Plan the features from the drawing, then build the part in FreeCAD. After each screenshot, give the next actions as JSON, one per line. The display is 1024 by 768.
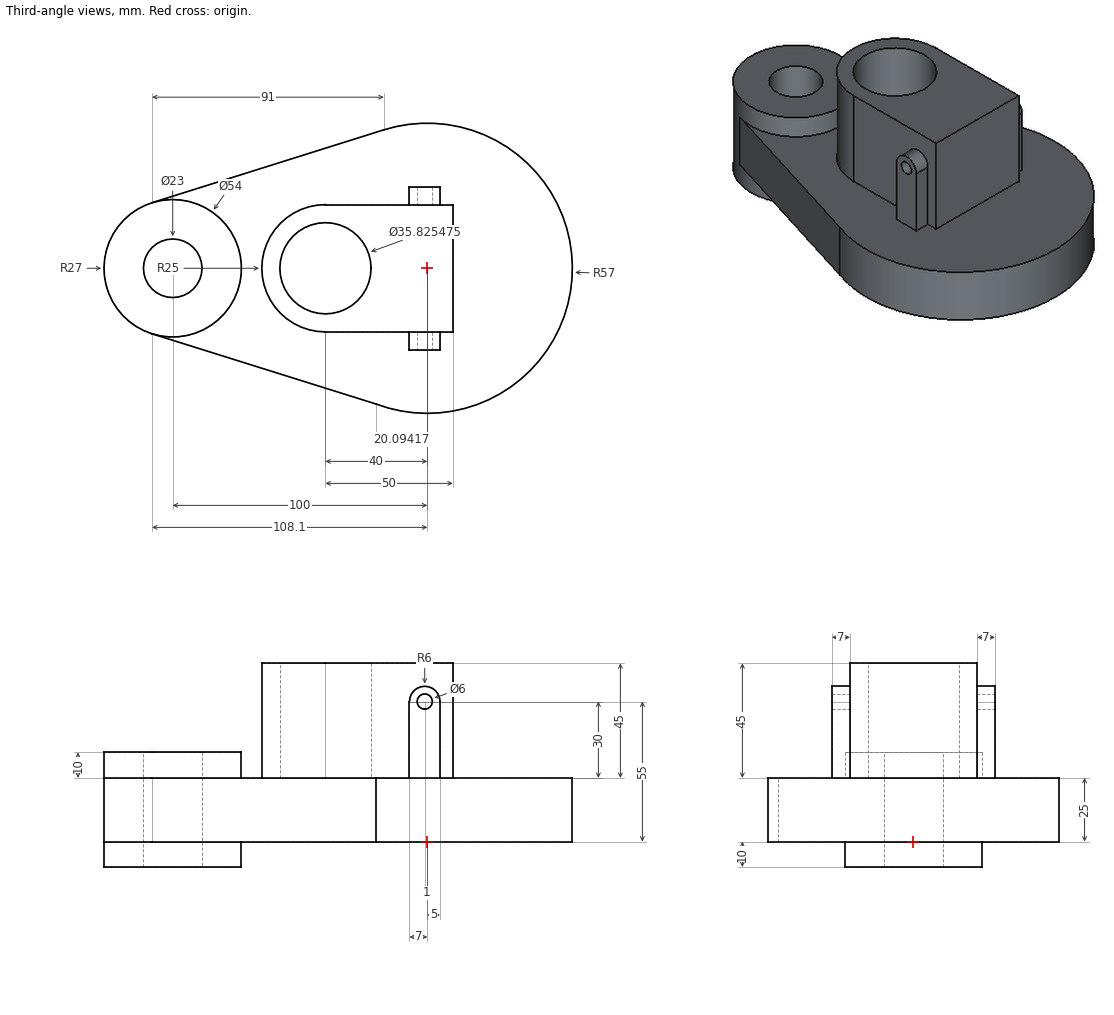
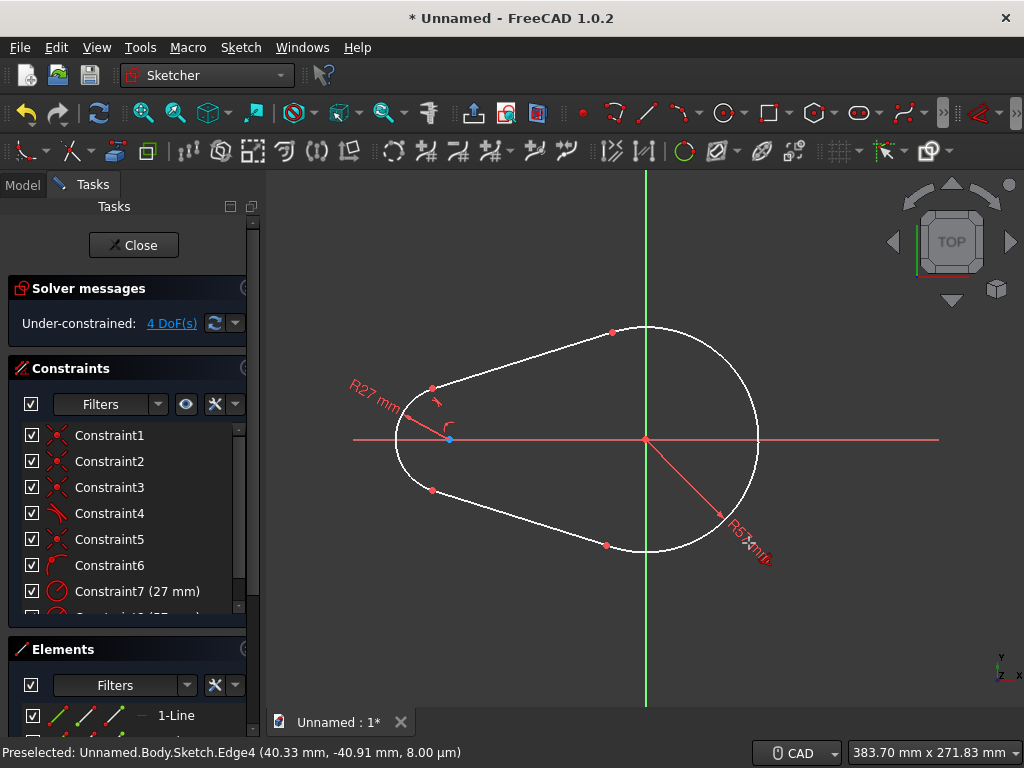
{"action": "left_click", "coordinate": [558, 349]}
{"action": "left_click", "coordinate": [523, 298]}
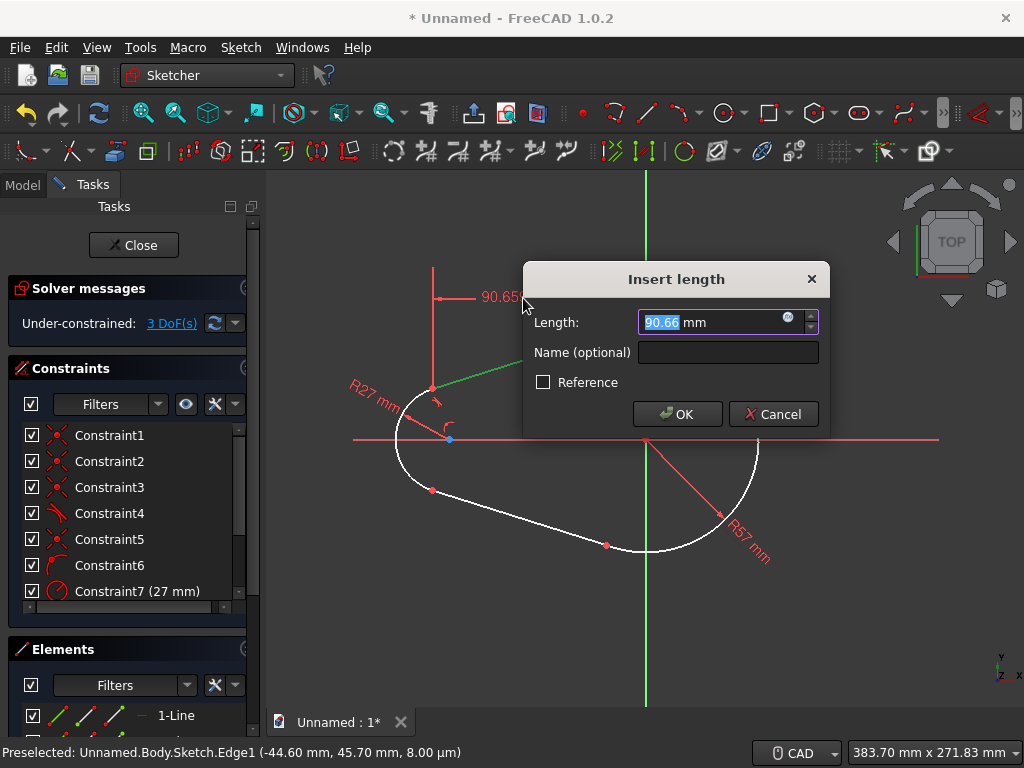
{"action": "type", "text": "91"}
{"action": "key", "text": "Return"}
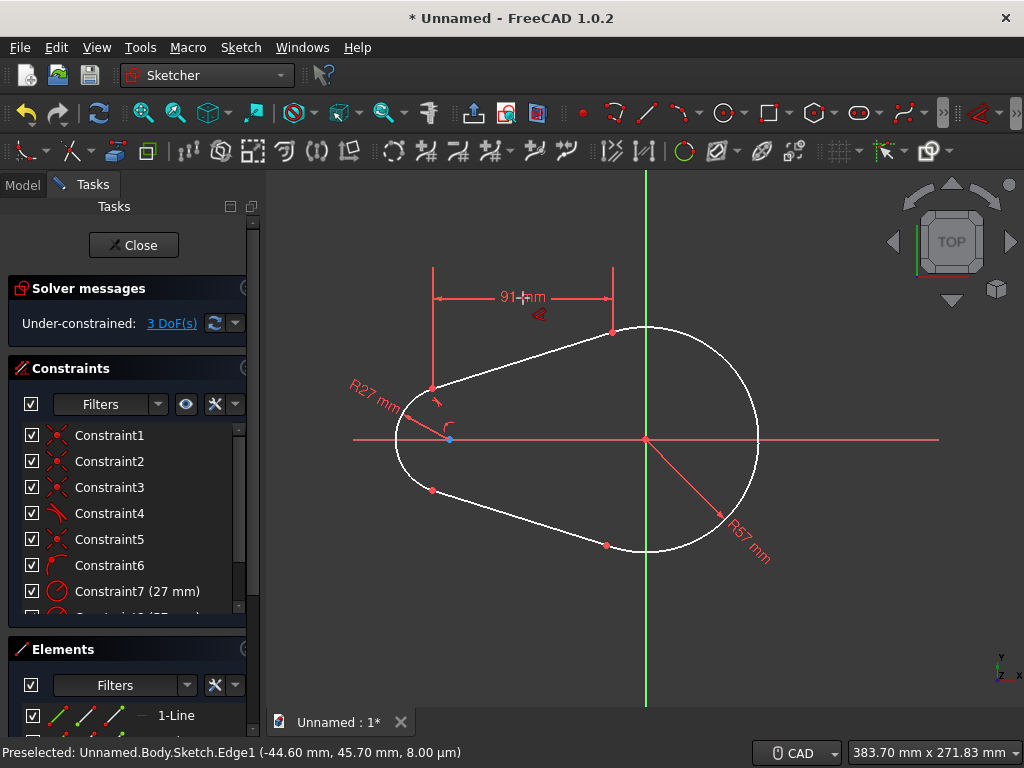
{"action": "left_click", "coordinate": [449, 440]}
{"action": "left_click", "coordinate": [547, 474]}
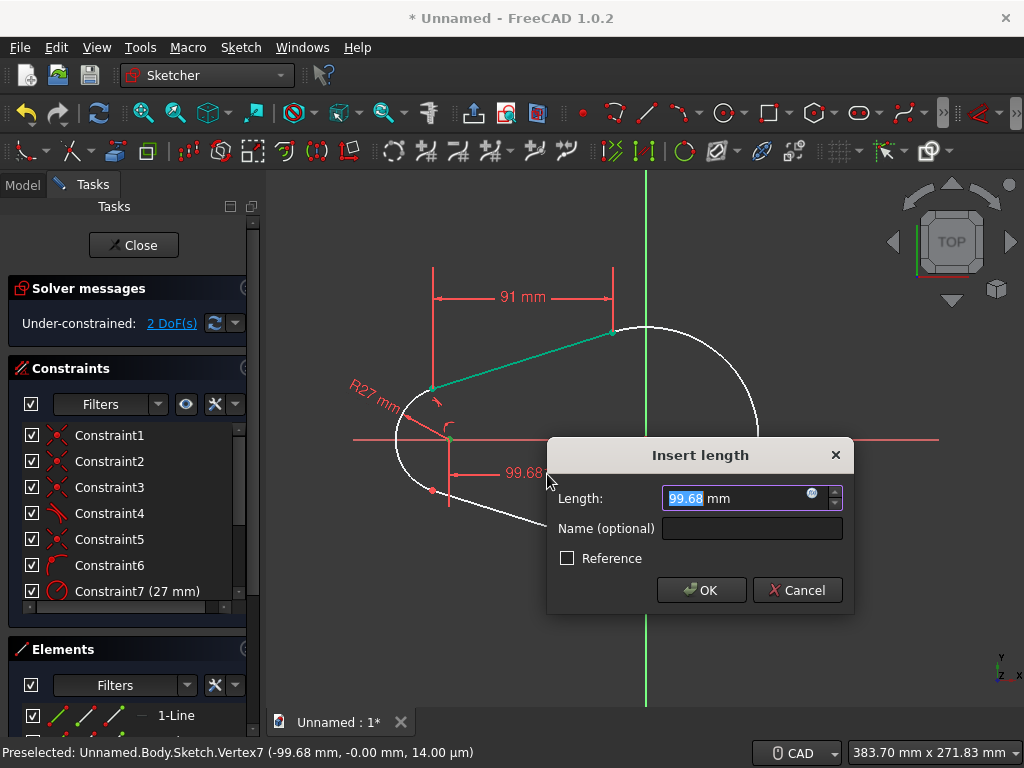
{"action": "type", "text": "100"}
{"action": "key", "text": "Return"}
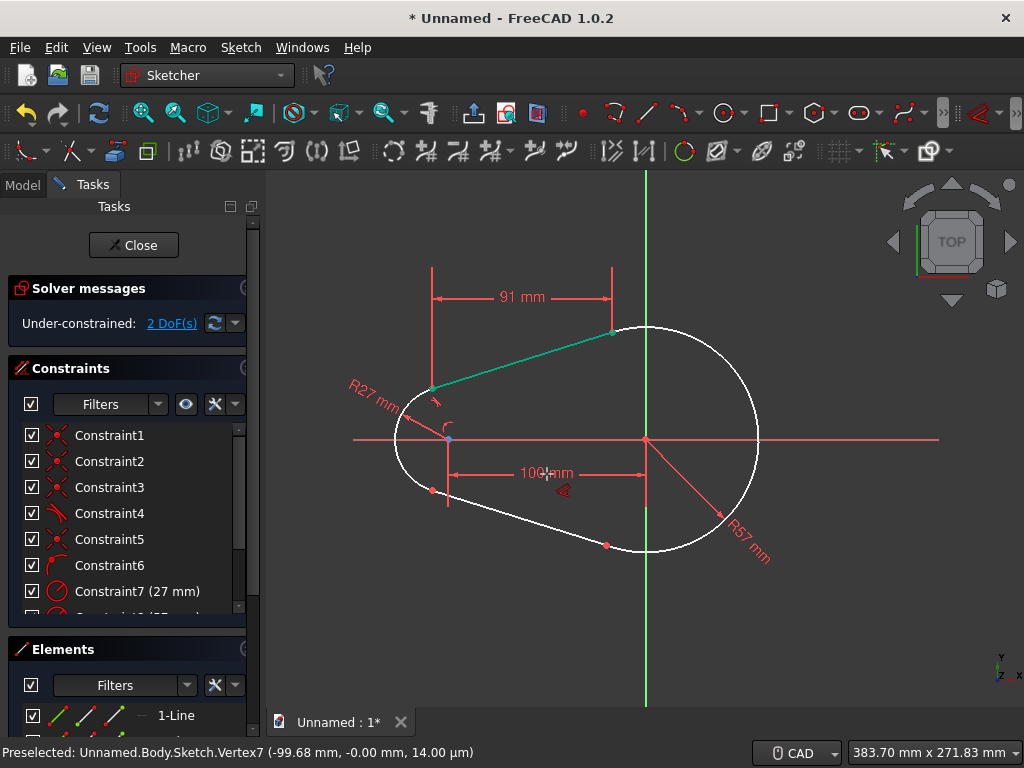
{"action": "left_click", "coordinate": [432, 491]}
{"action": "left_click", "coordinate": [490, 525]}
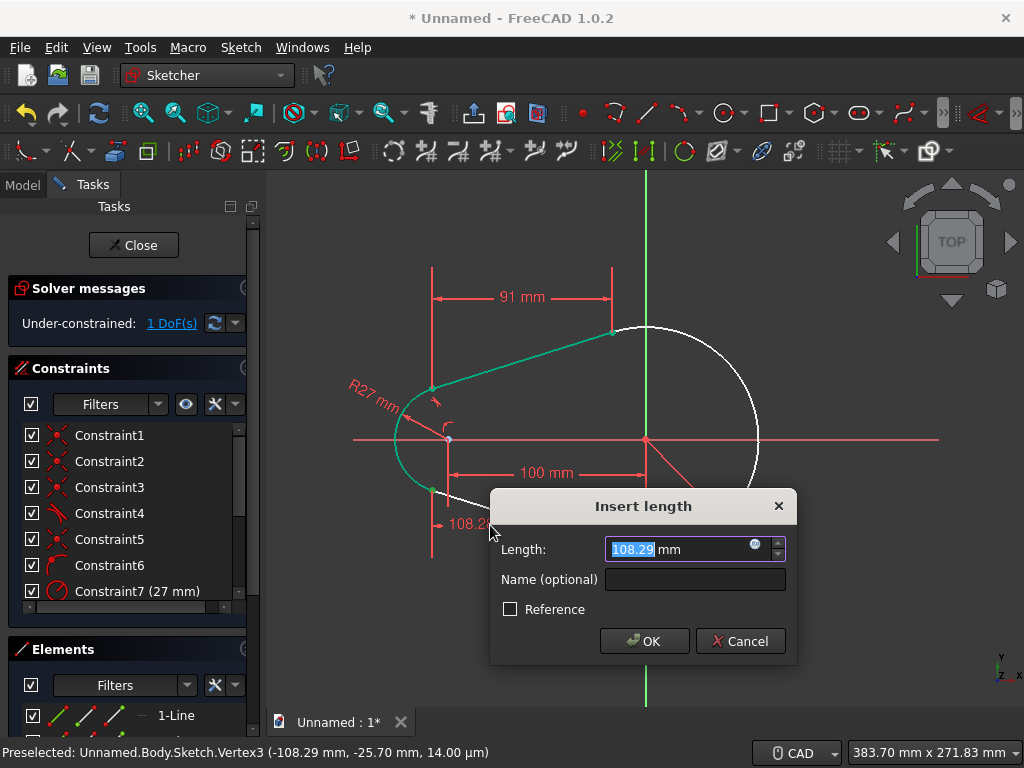
{"action": "type", "text": "108.1"}
{"action": "key", "text": "Return"}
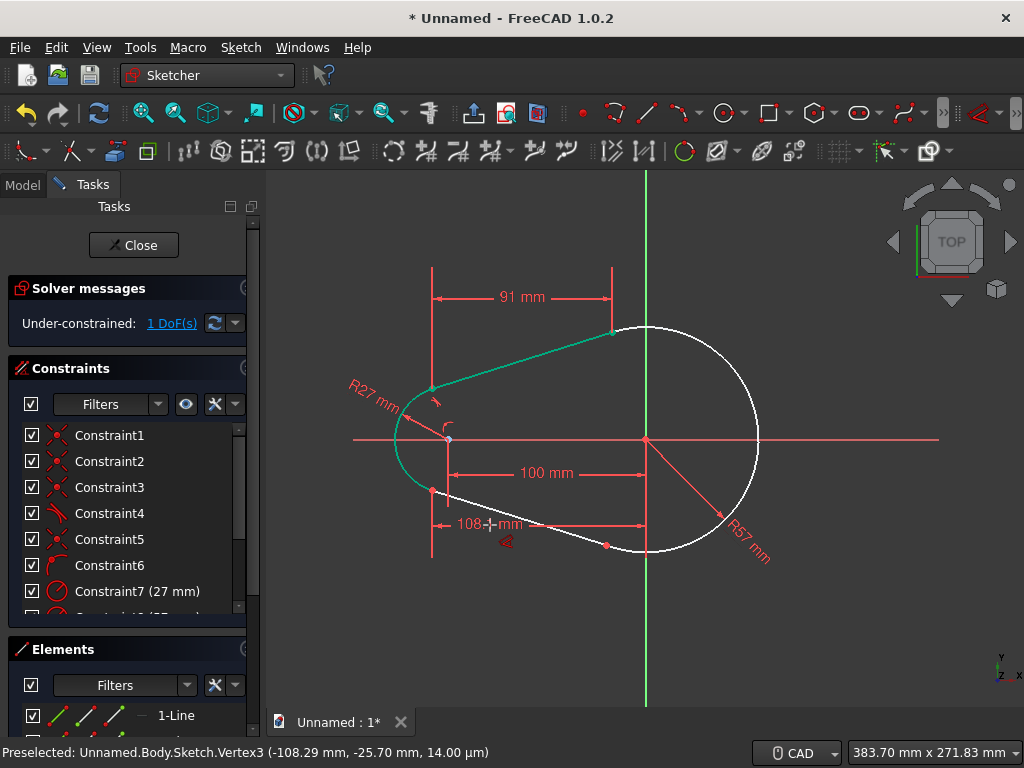
{"action": "left_click", "coordinate": [606, 545]}
{"action": "left_click", "coordinate": [626, 579]}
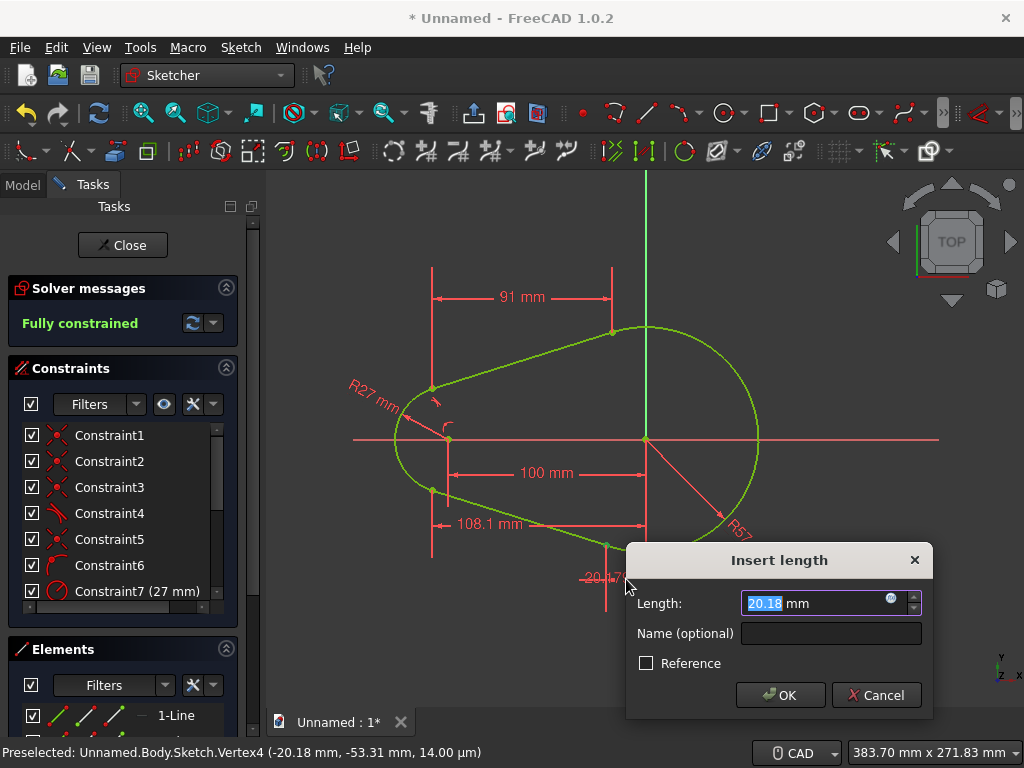
{"action": "type", "text": "20.09417"}
{"action": "key", "text": "Return"}
{"action": "key", "text": "Escape"}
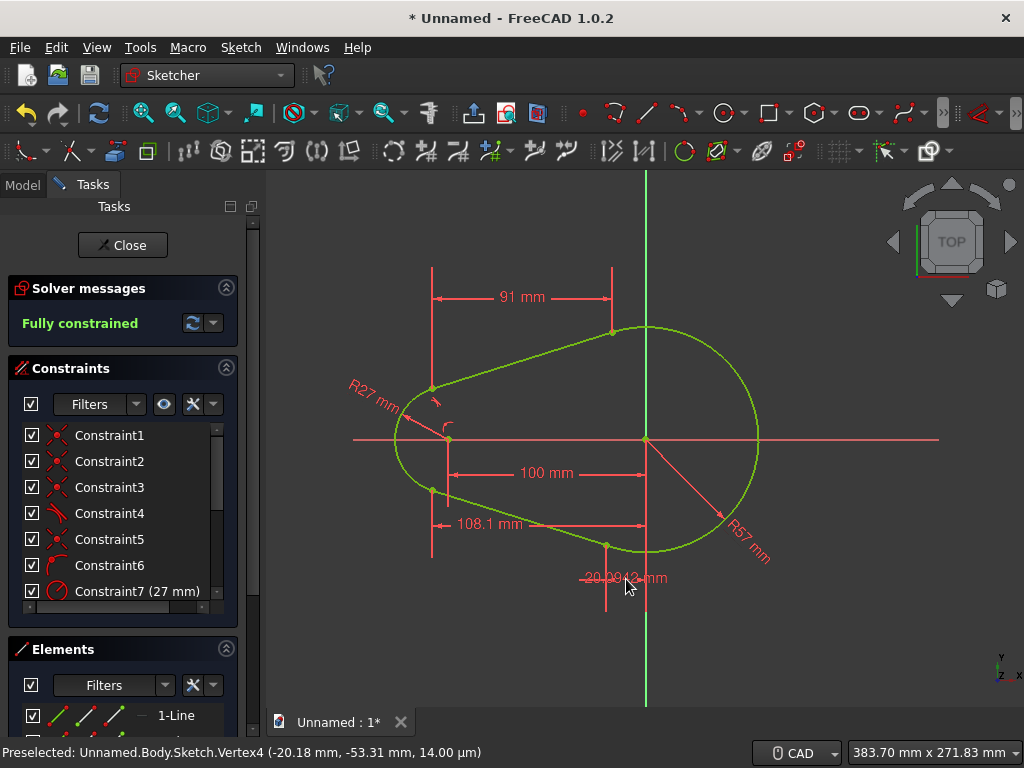
{"action": "left_click", "coordinate": [123, 245]}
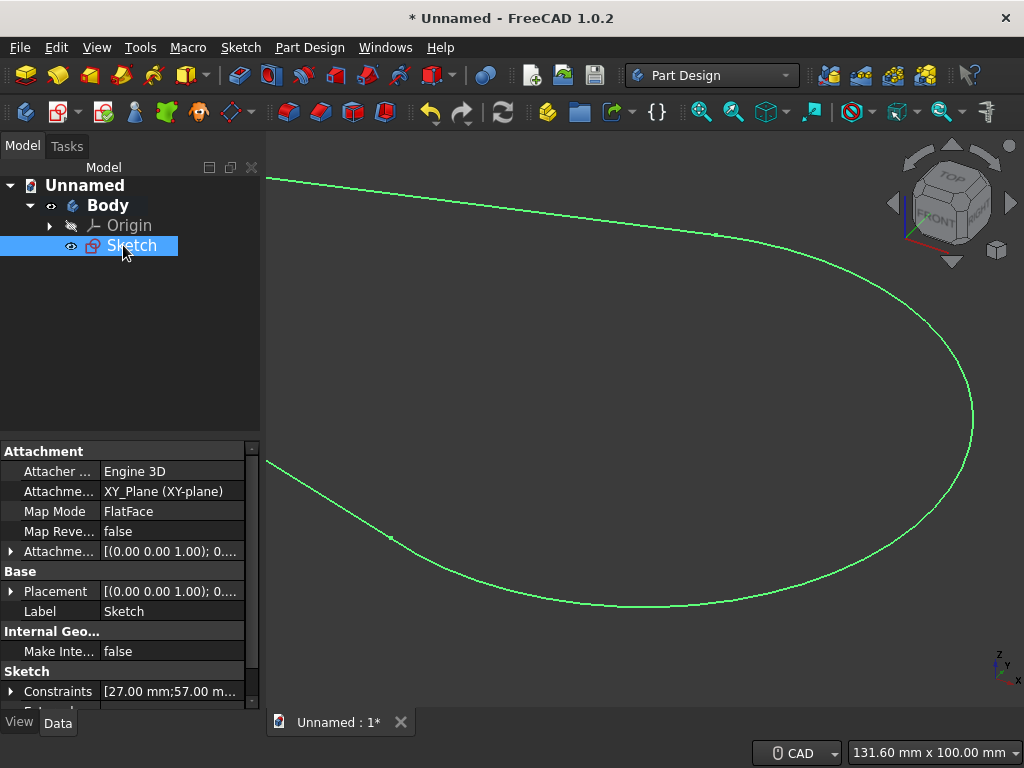
{"action": "left_click", "coordinate": [26, 76]}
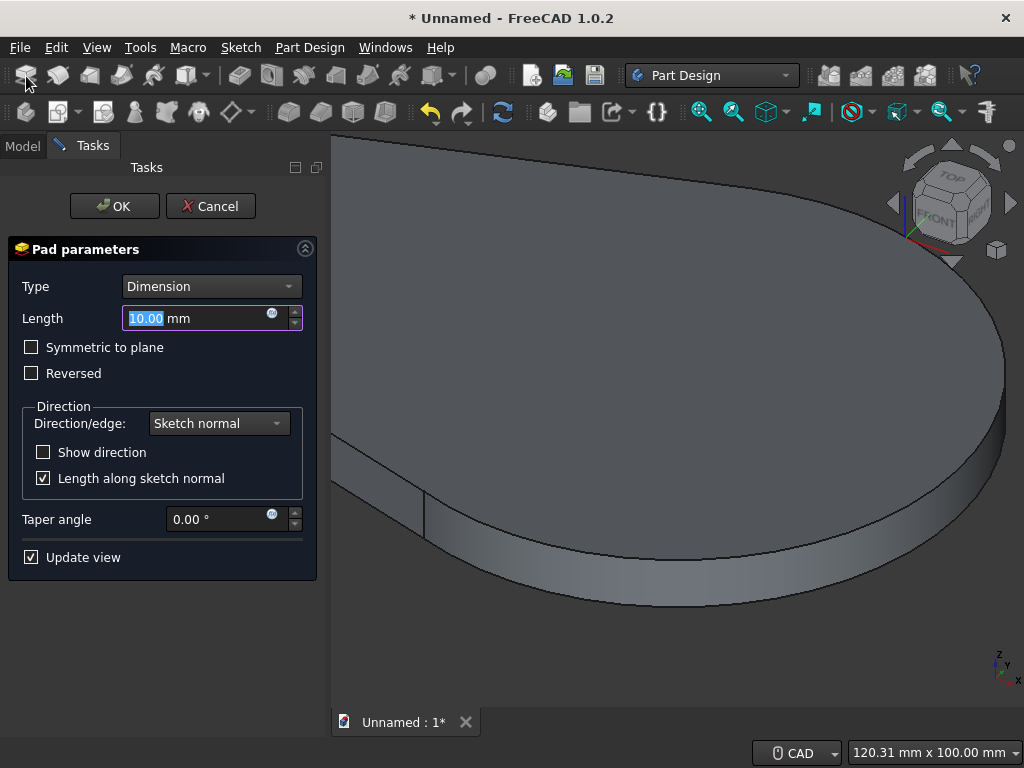
{"action": "type", "text": "25"}
{"action": "key", "text": "Tab"}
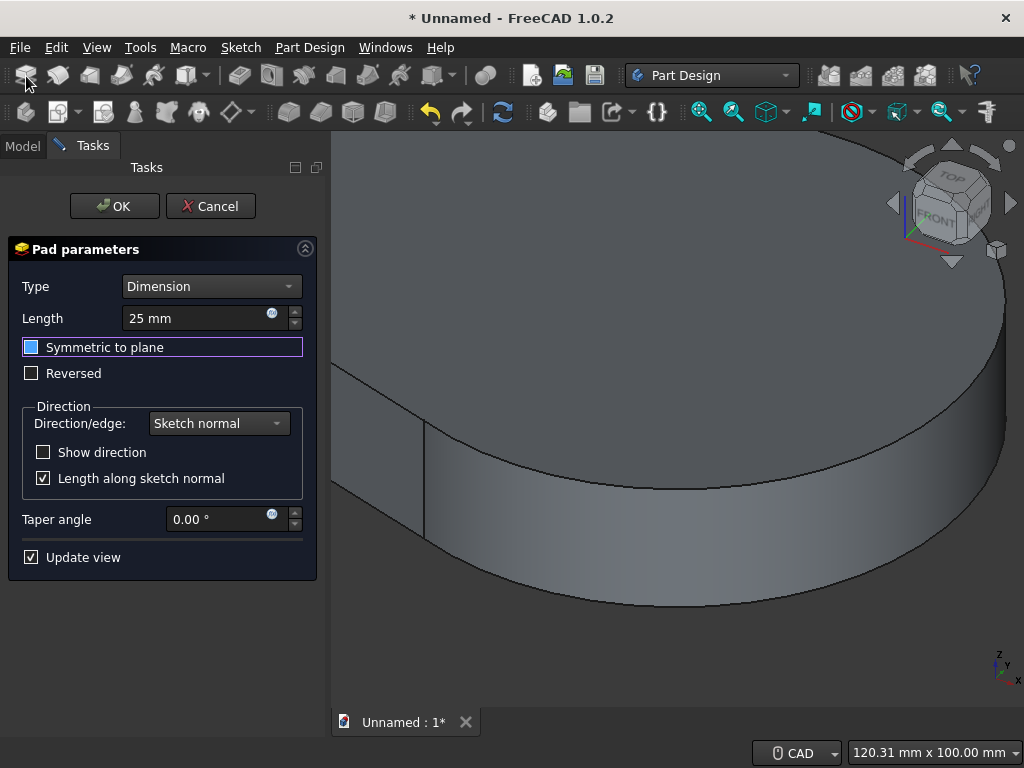
{"action": "left_click", "coordinate": [115, 206]}